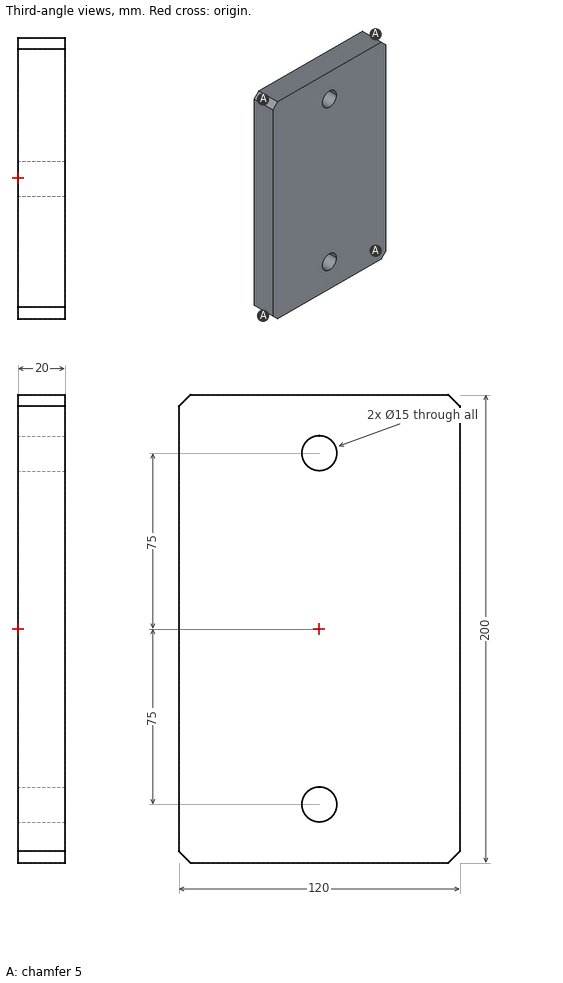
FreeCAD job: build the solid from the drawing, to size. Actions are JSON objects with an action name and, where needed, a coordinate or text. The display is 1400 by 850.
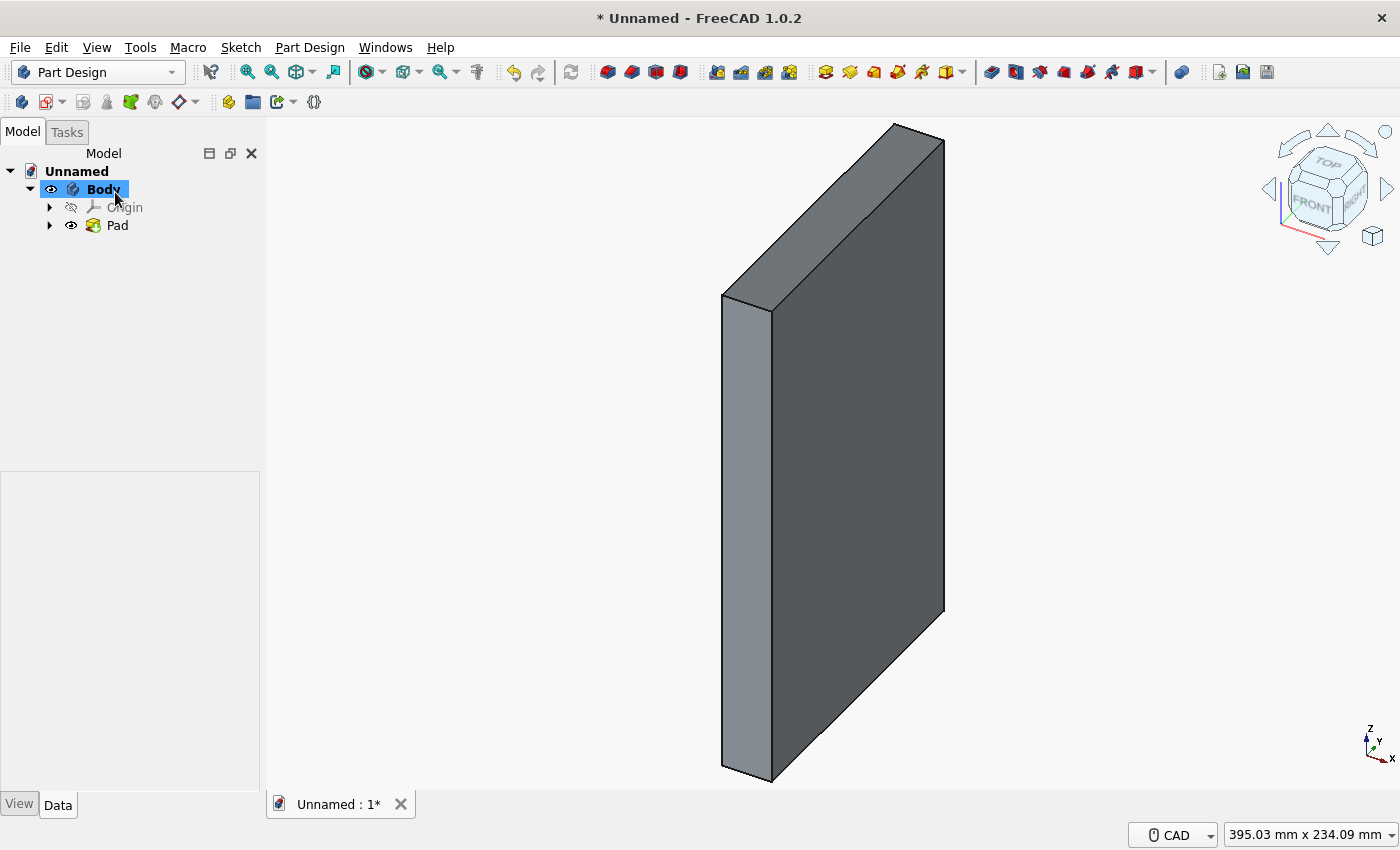
{"action": "left_click", "coordinate": [858, 460]}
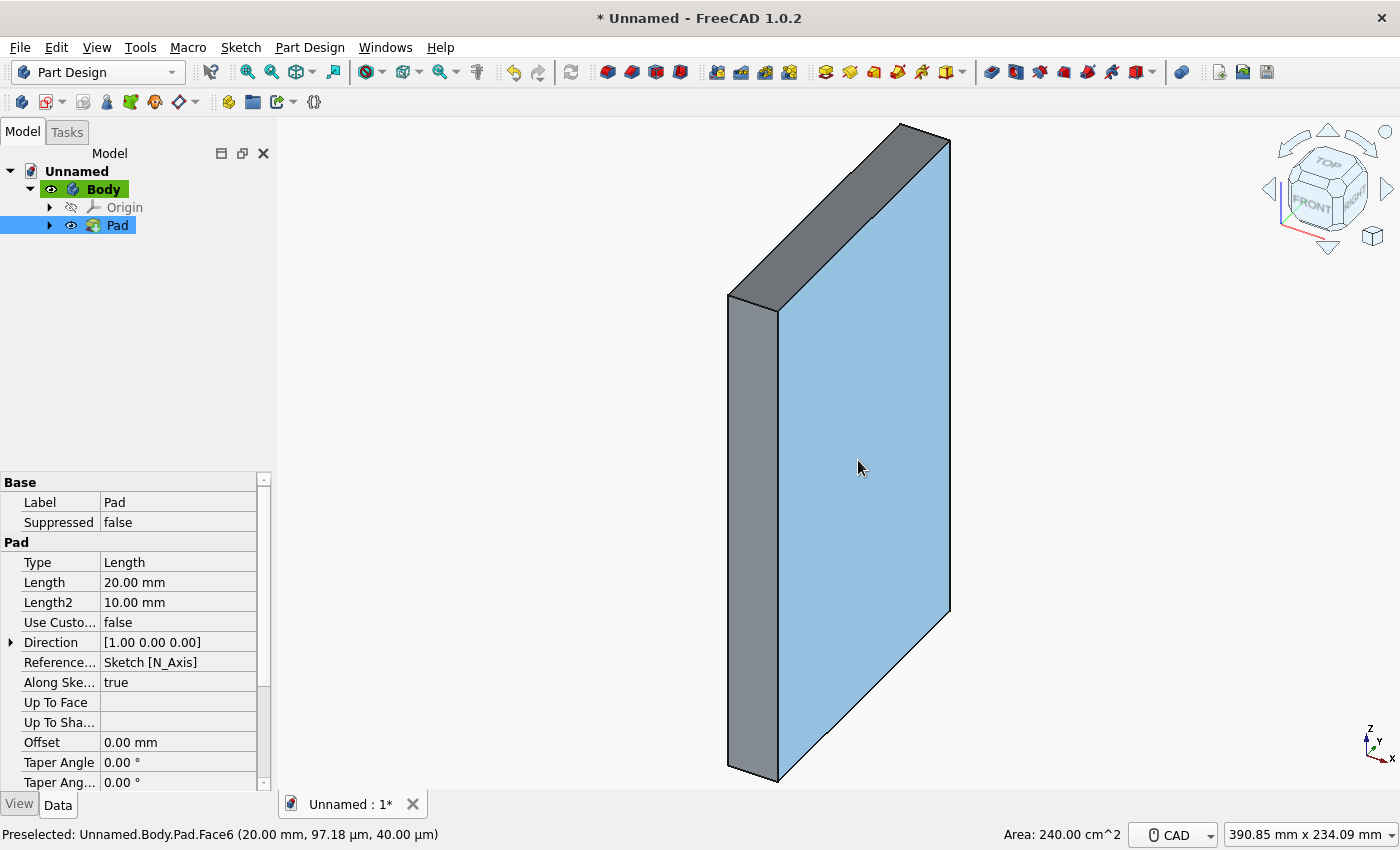
{"action": "left_click", "coordinate": [46, 102]}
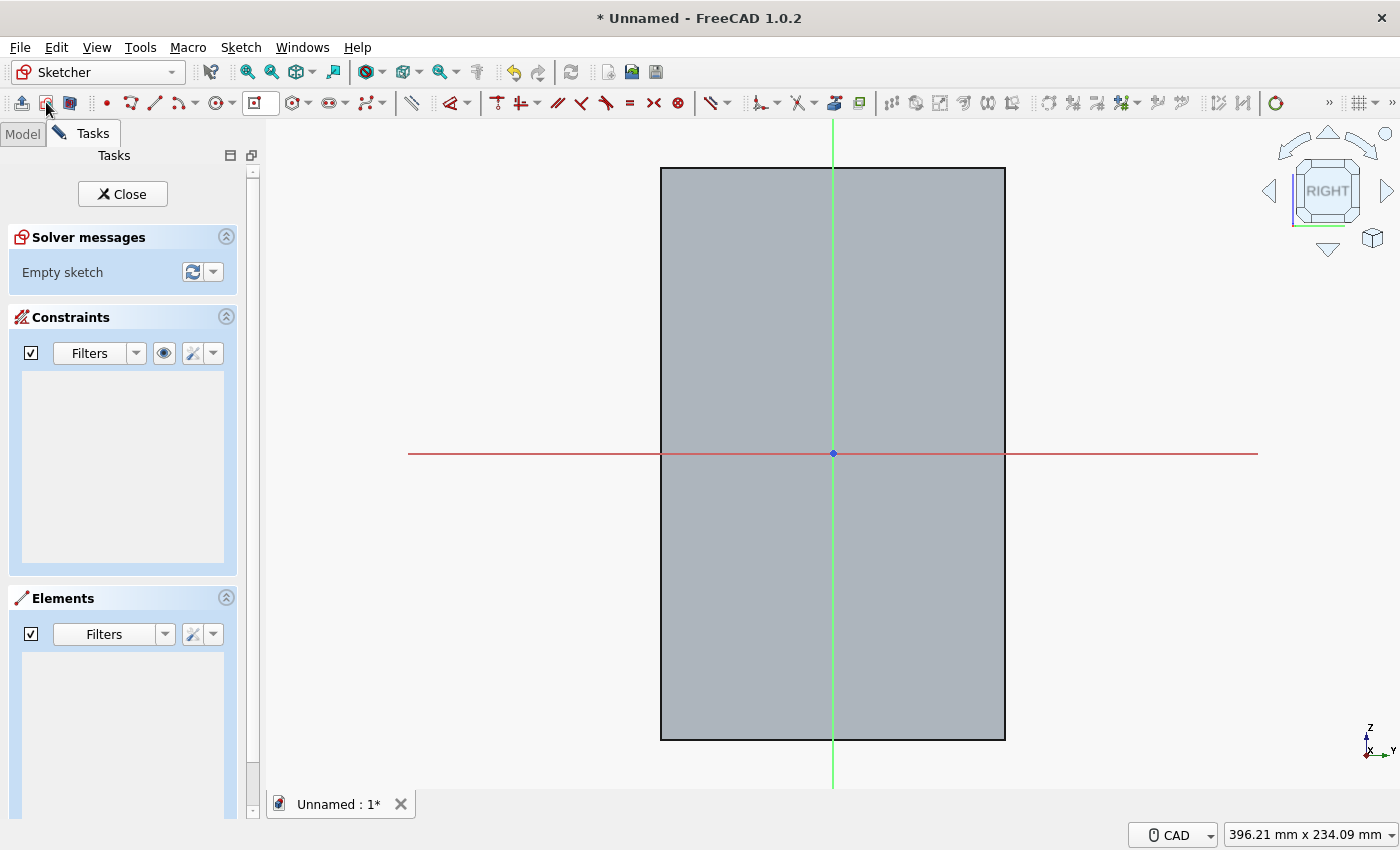
{"action": "key", "text": "g c"}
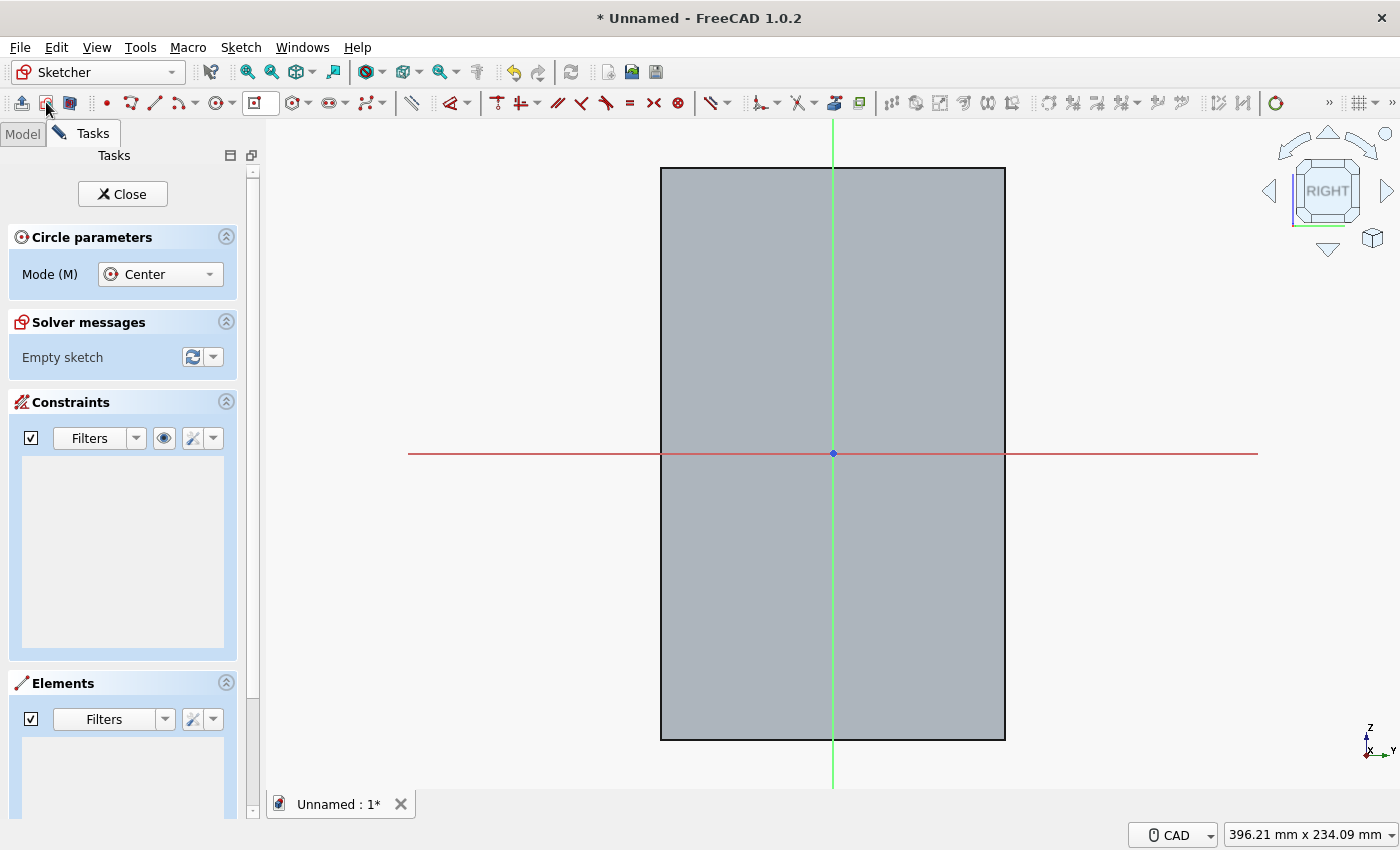
{"action": "left_click", "coordinate": [833, 239]}
{"action": "left_click", "coordinate": [848, 224]}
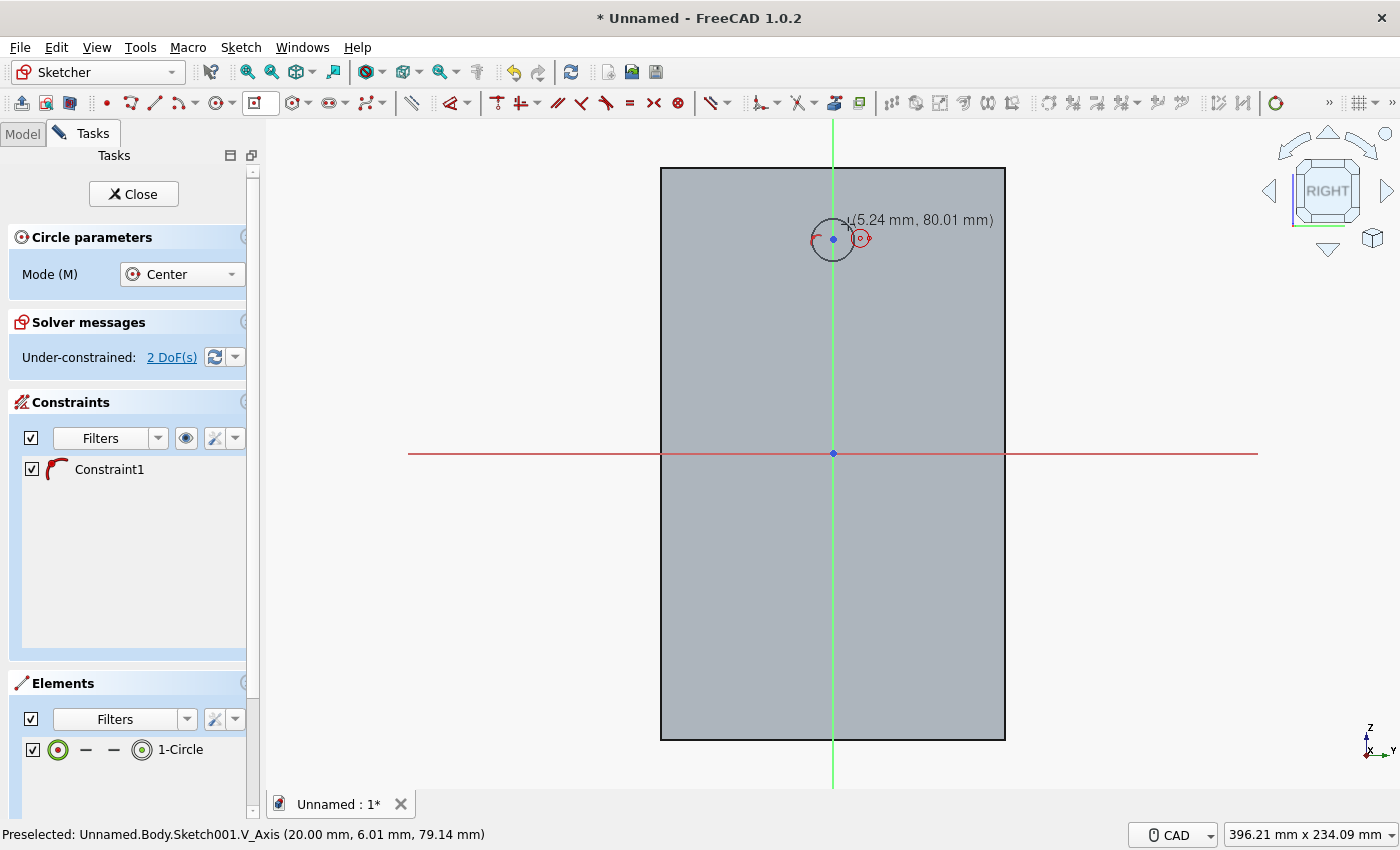
{"action": "left_click", "coordinate": [833, 669]}
{"action": "left_click", "coordinate": [848, 653]}
{"action": "key", "text": "Escape"}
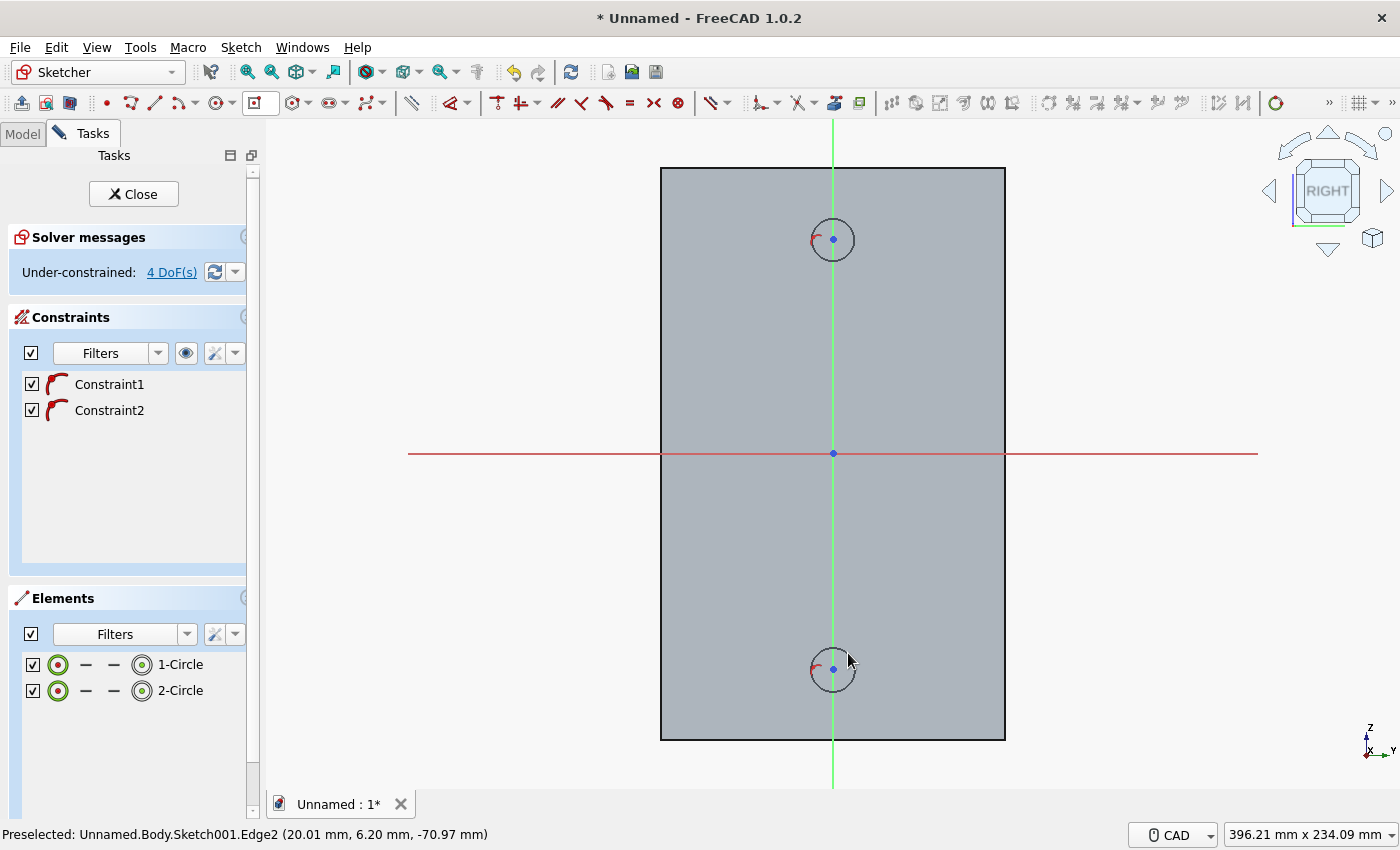
{"action": "left_click", "coordinate": [848, 225]}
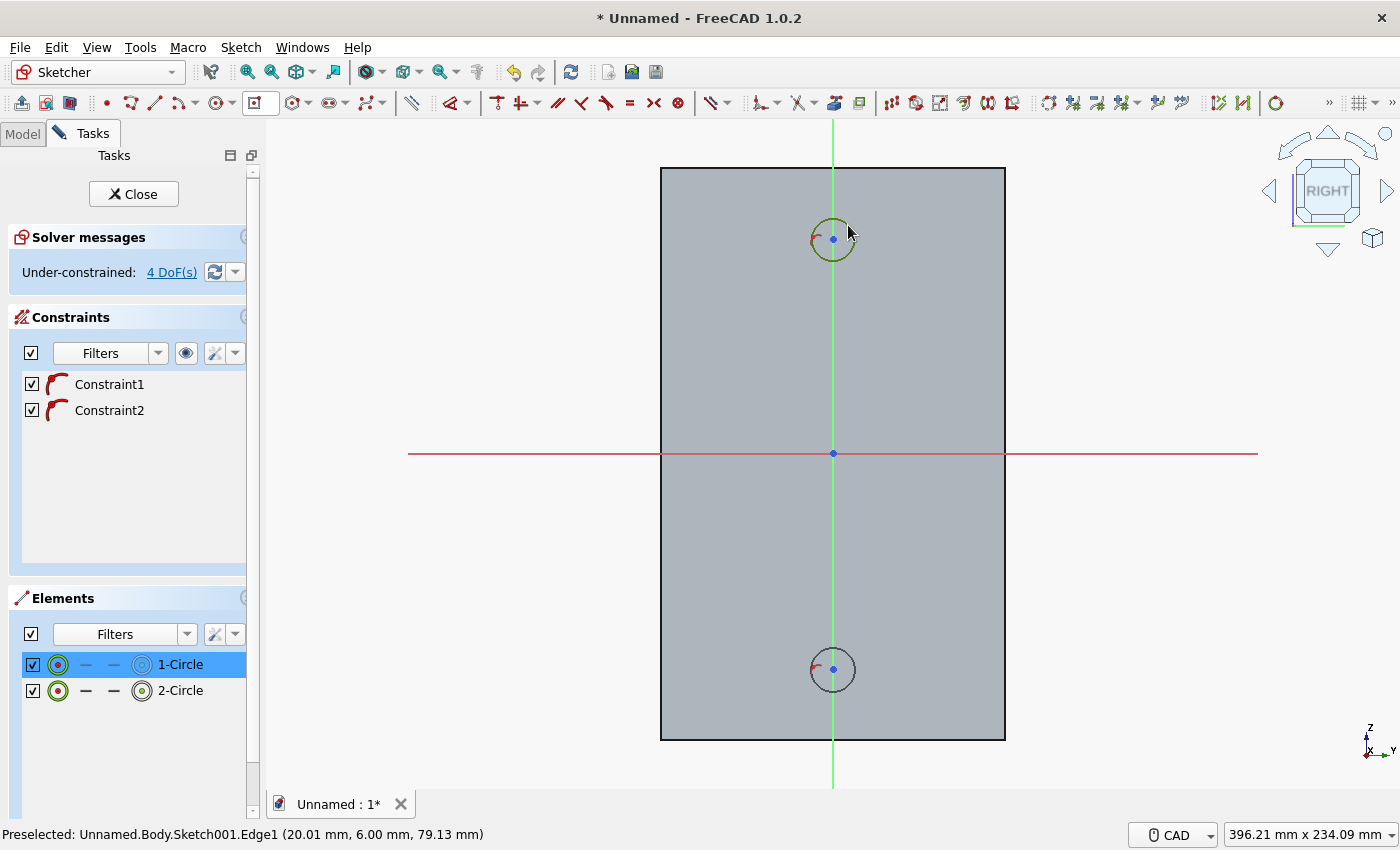
{"action": "left_click", "coordinate": [848, 654]}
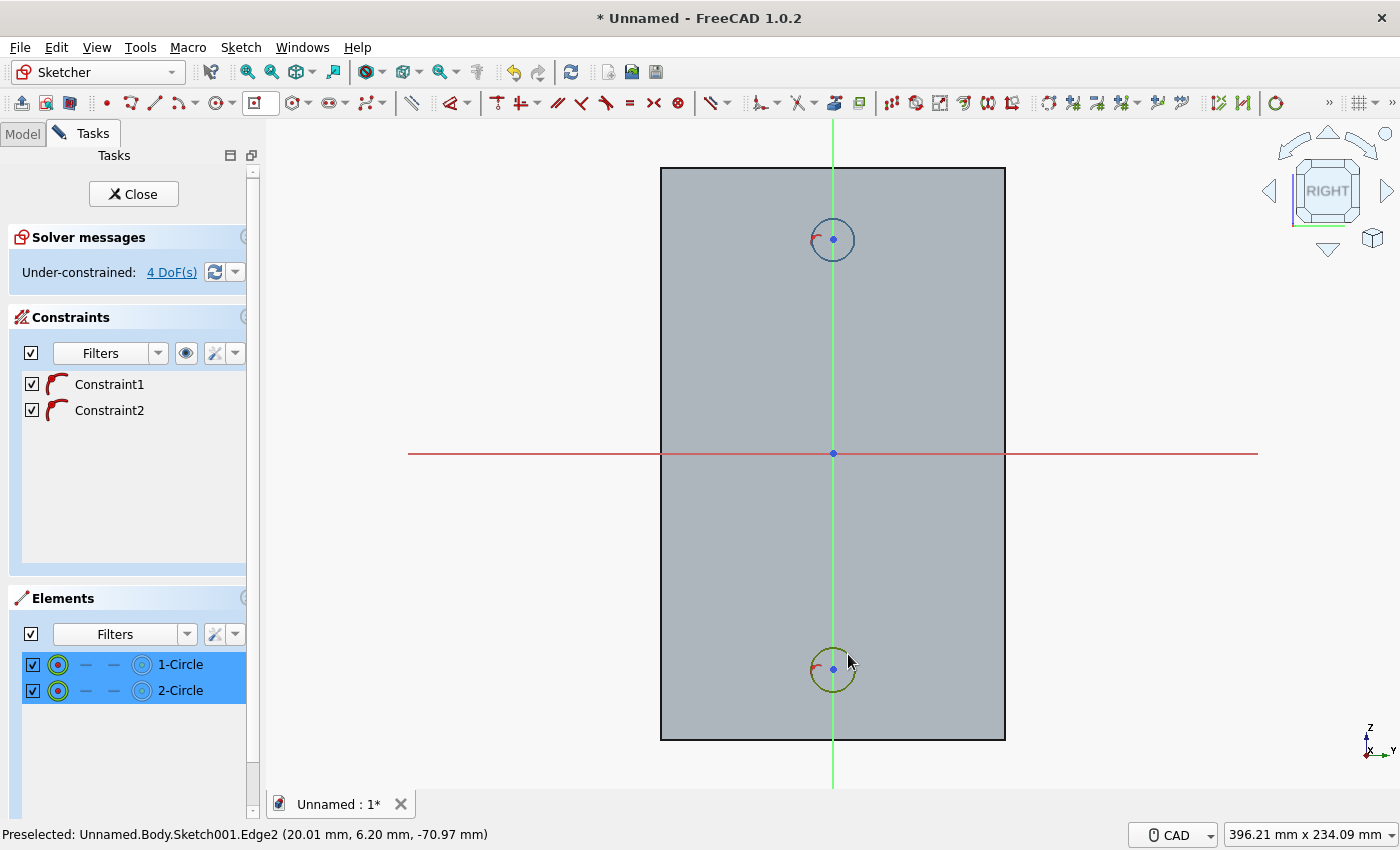
{"action": "key", "text": "e"}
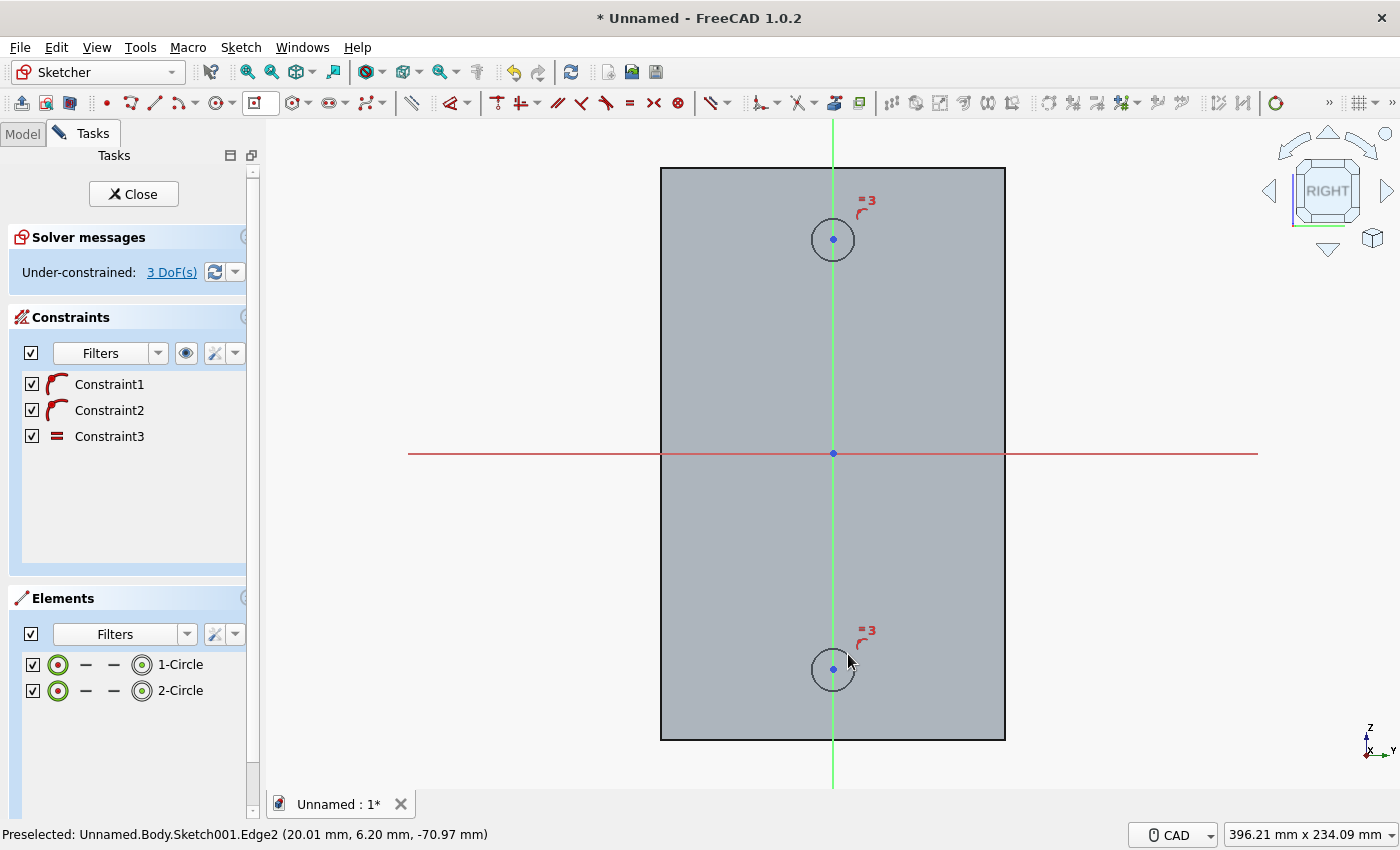
{"action": "key", "text": "d"}